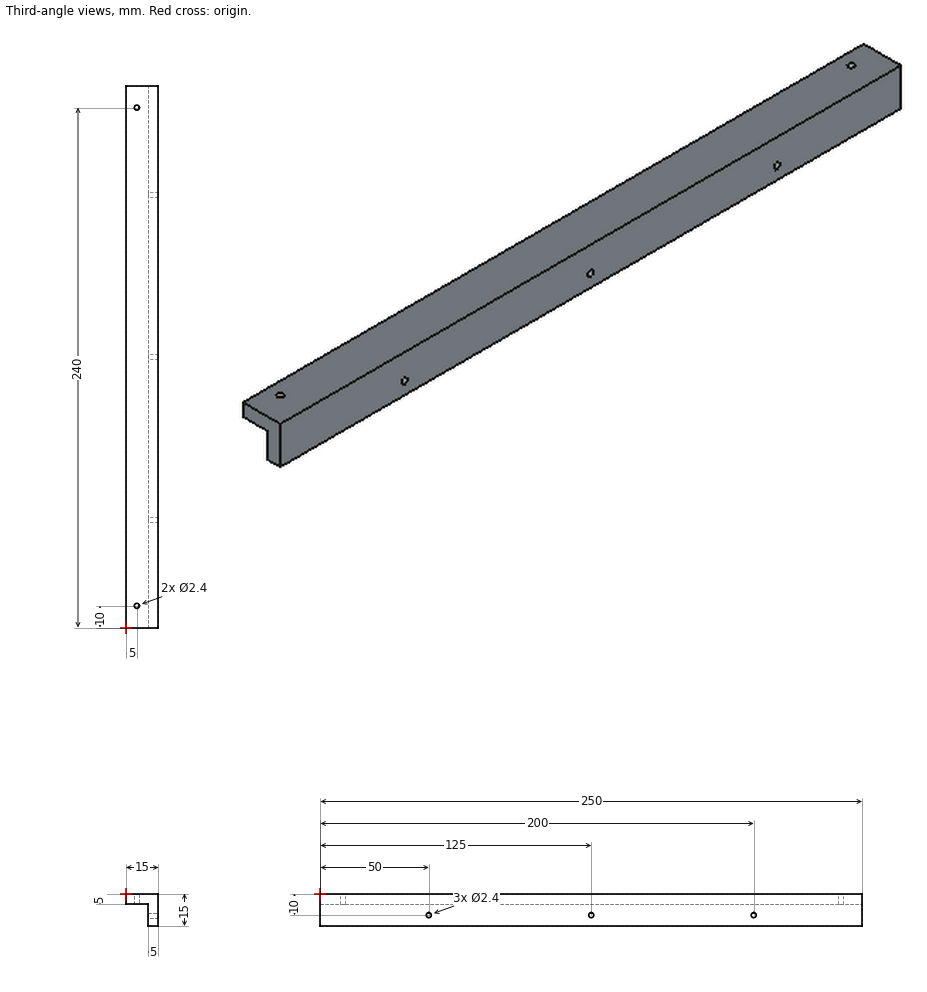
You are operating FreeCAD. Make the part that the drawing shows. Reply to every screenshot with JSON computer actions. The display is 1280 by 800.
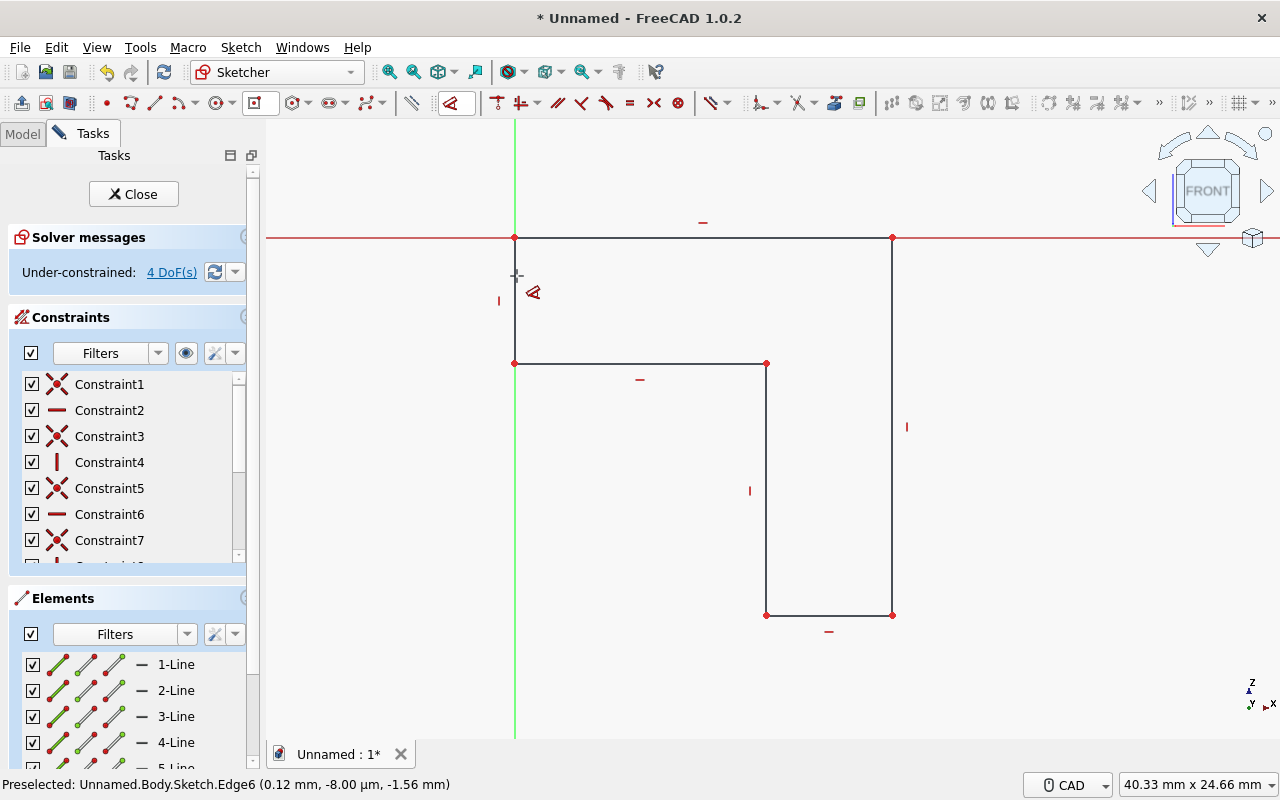
{"action": "left_click", "coordinate": [854, 616]}
{"action": "left_click", "coordinate": [829, 650]}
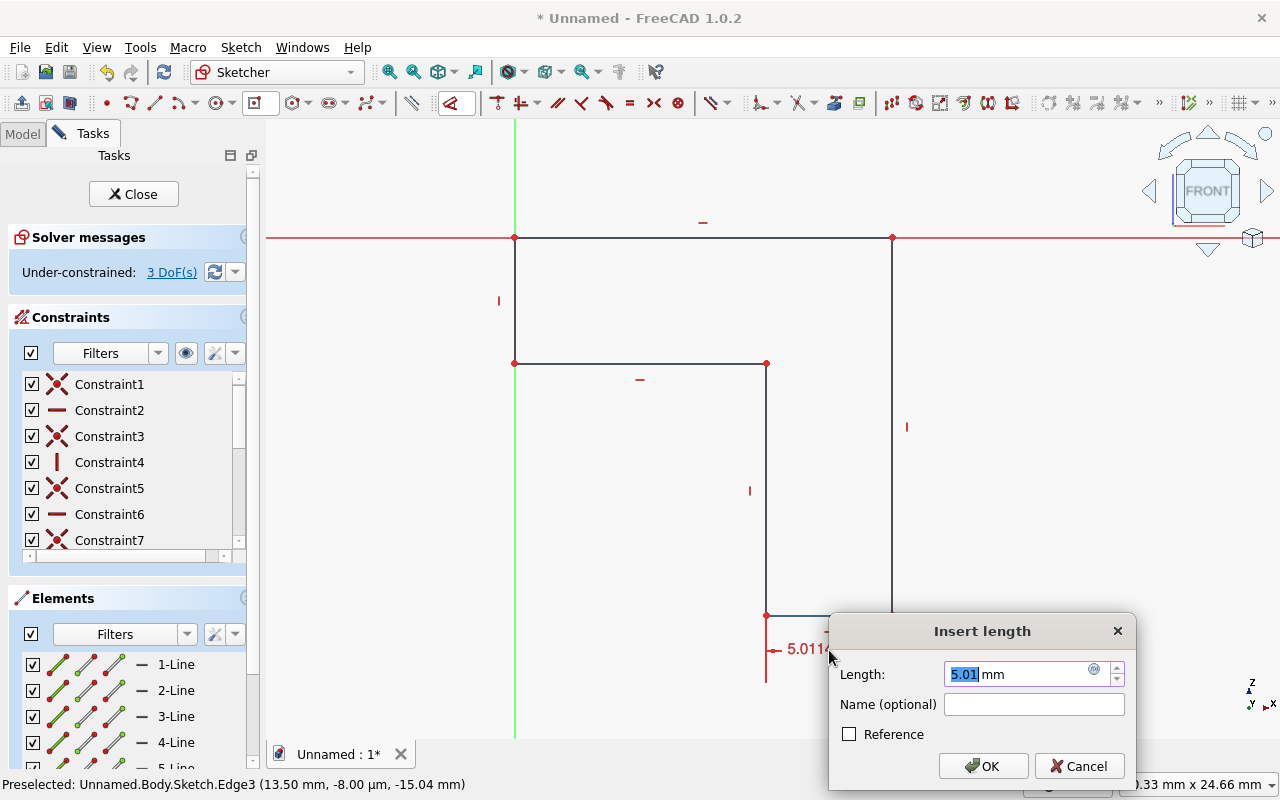
{"action": "type", "text": "5"}
{"action": "key", "text": "Return"}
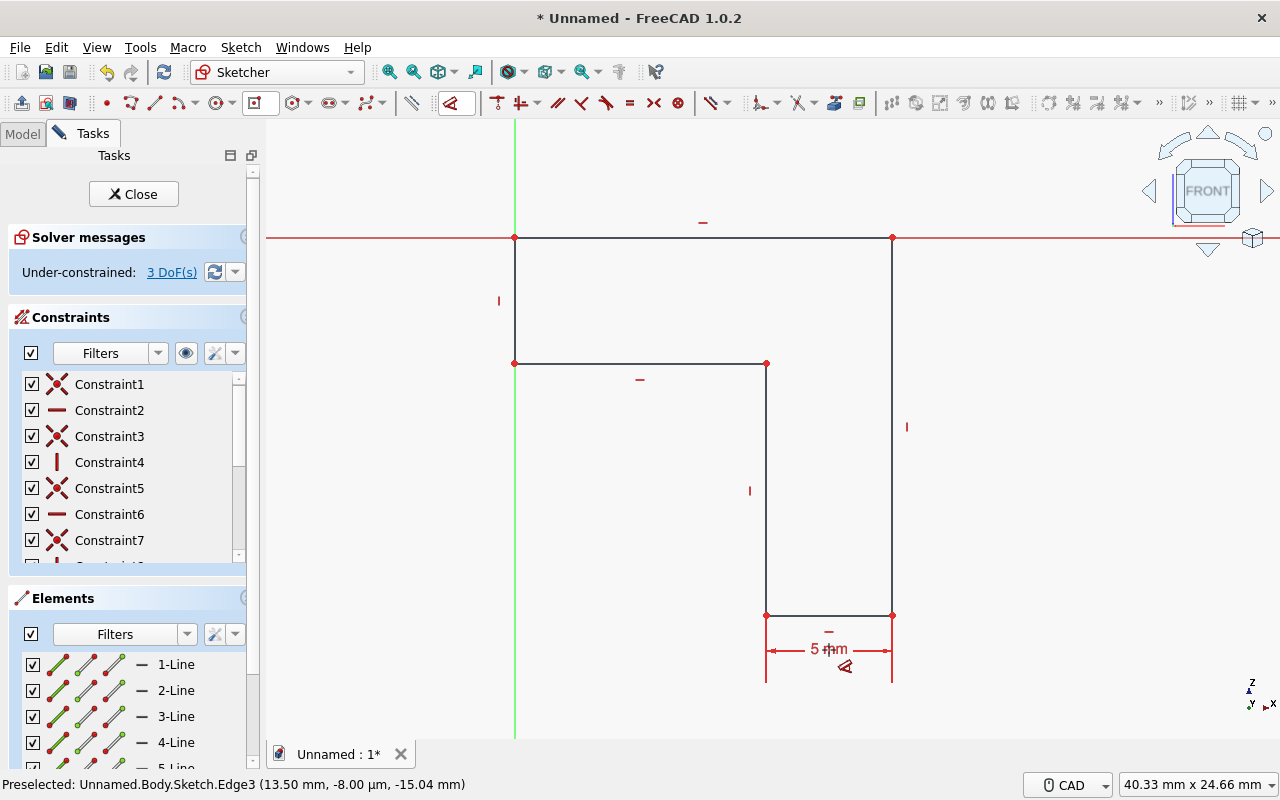
{"action": "left_click", "coordinate": [515, 326]}
{"action": "left_click", "coordinate": [481, 301]}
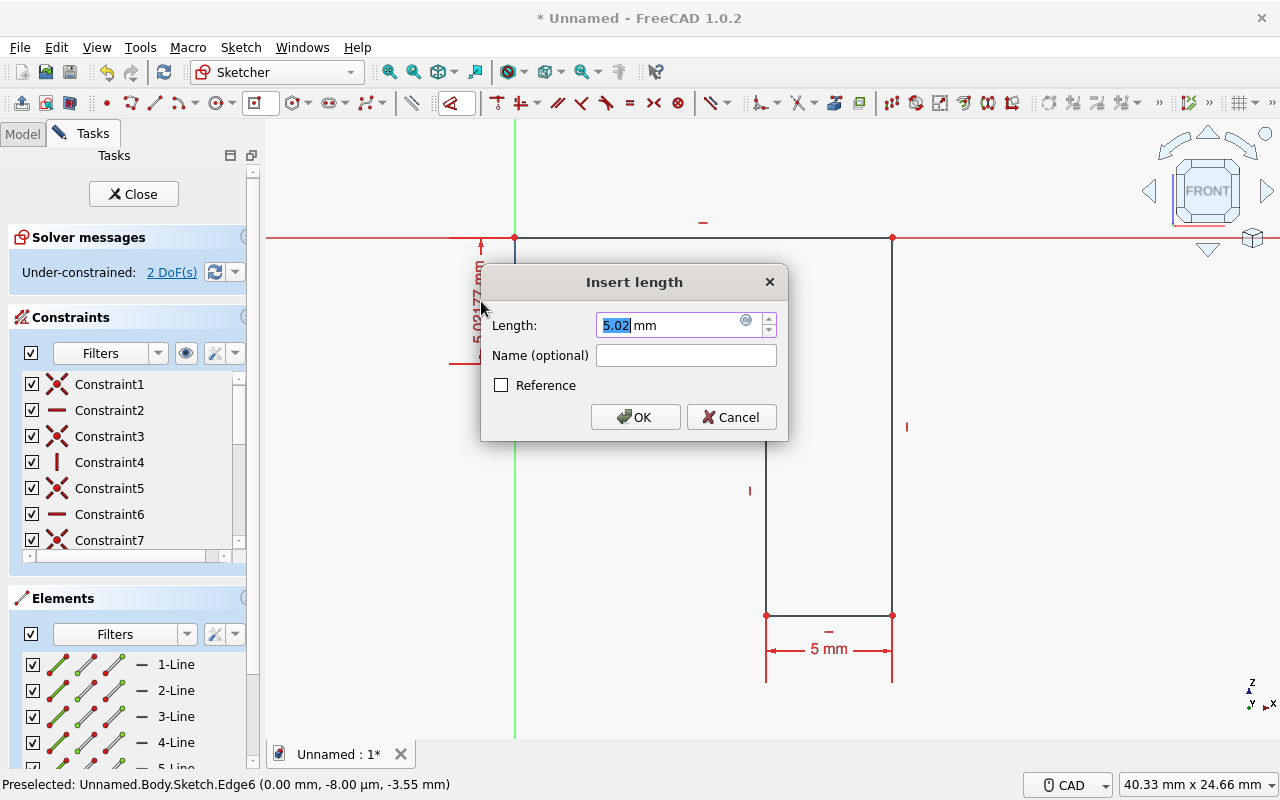
{"action": "type", "text": "5"}
{"action": "key", "text": "Return"}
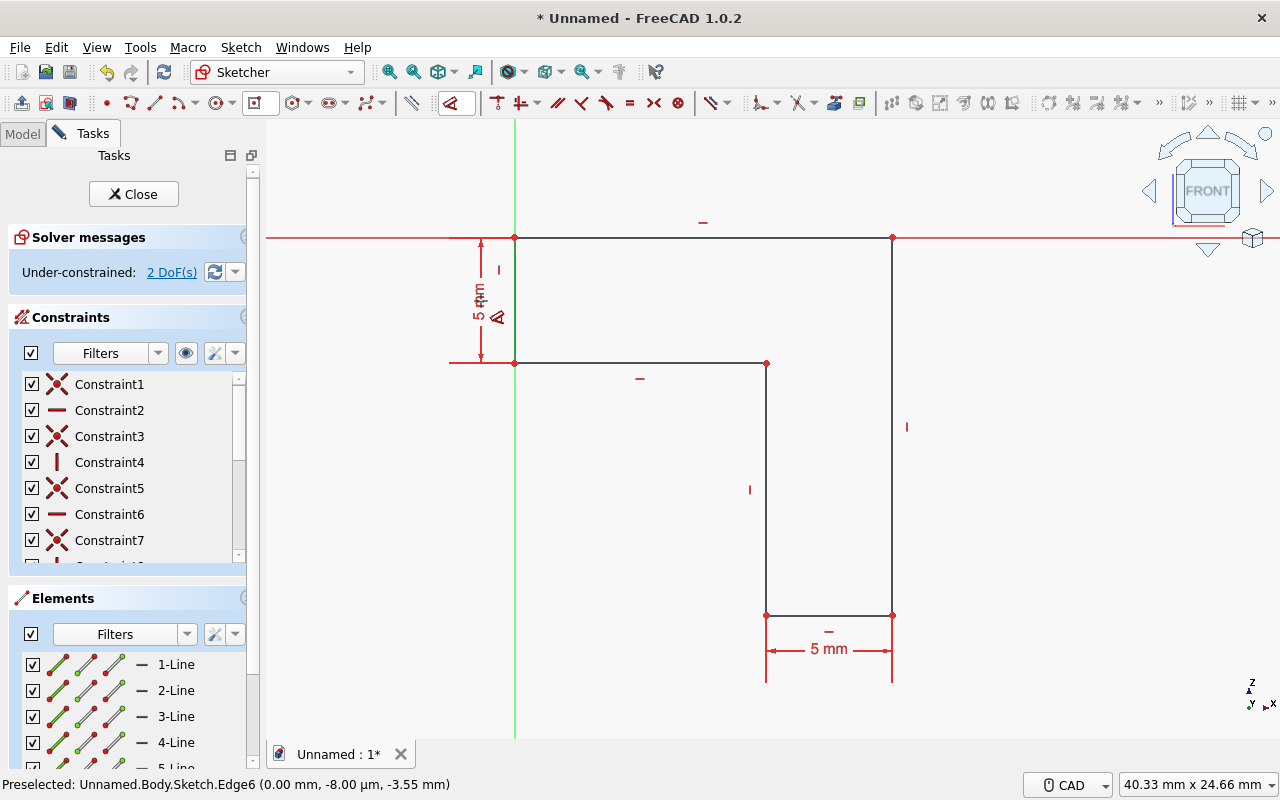
{"action": "left_click", "coordinate": [628, 238]}
{"action": "left_click", "coordinate": [703, 204]}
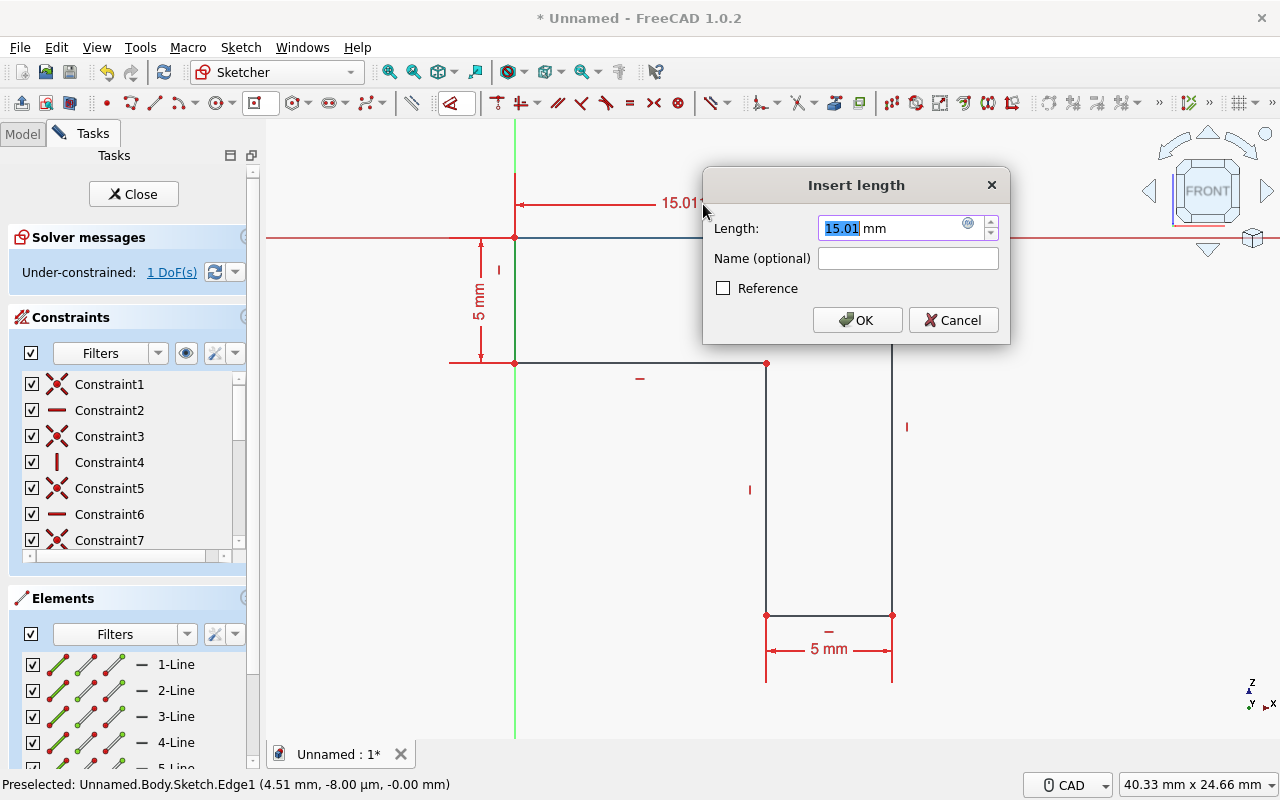
{"action": "type", "text": "15"}
{"action": "key", "text": "Return"}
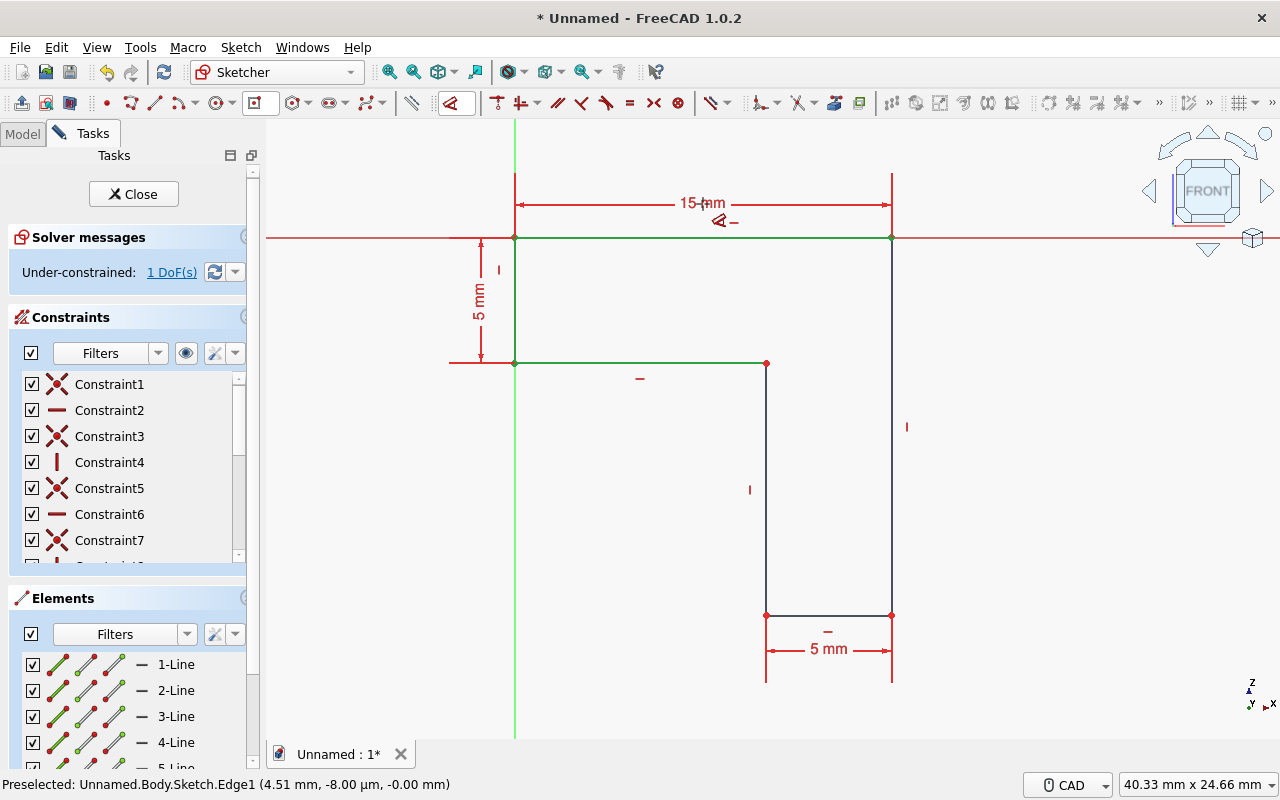
{"action": "left_click", "coordinate": [892, 351]}
{"action": "left_click", "coordinate": [926, 427]}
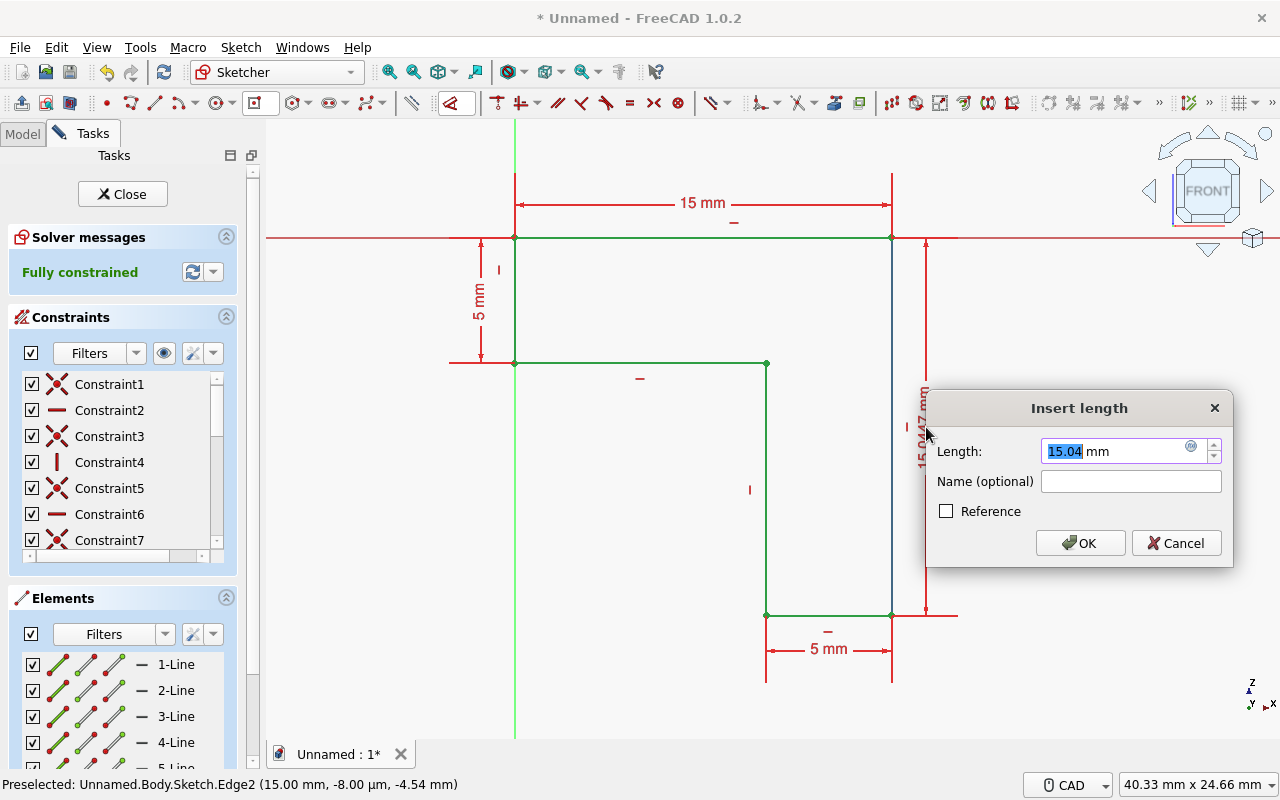
{"action": "type", "text": "15"}
{"action": "key", "text": "Return"}
{"action": "key", "text": "Escape"}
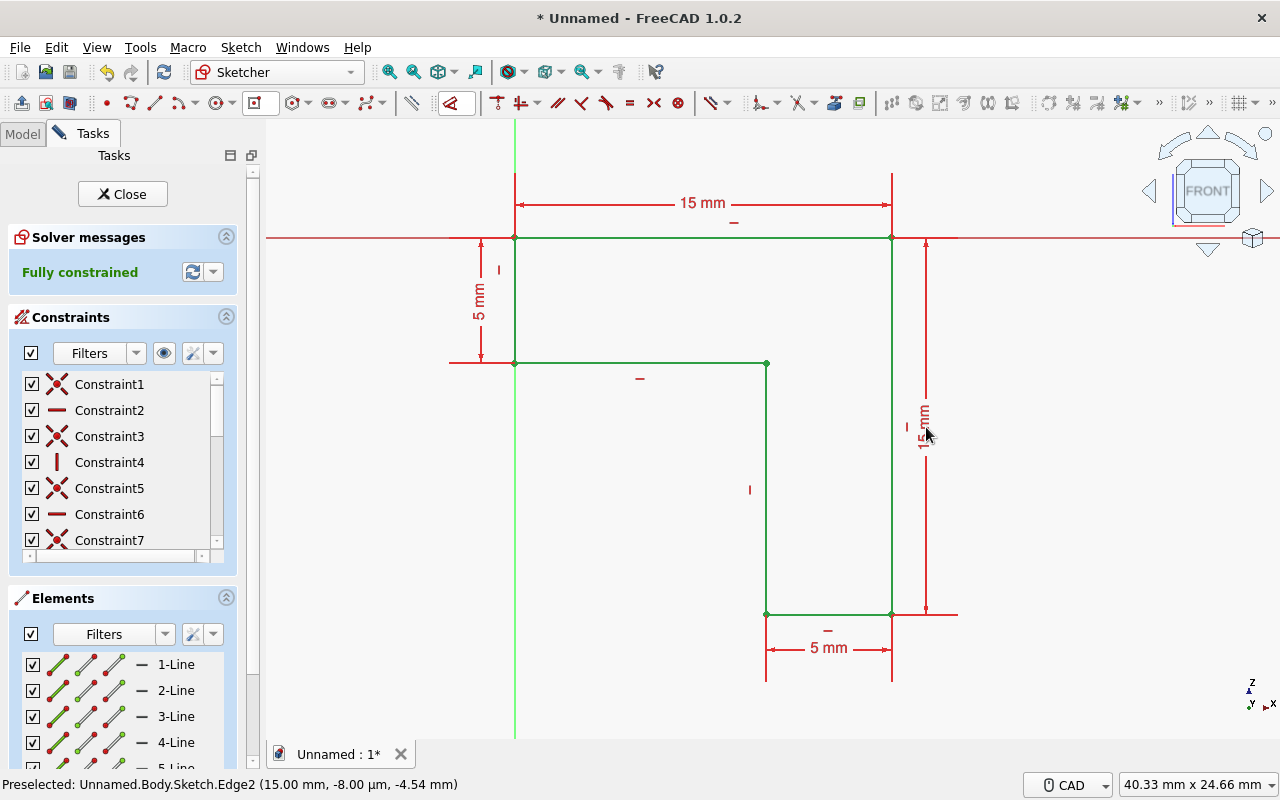
{"action": "left_click", "coordinate": [123, 194]}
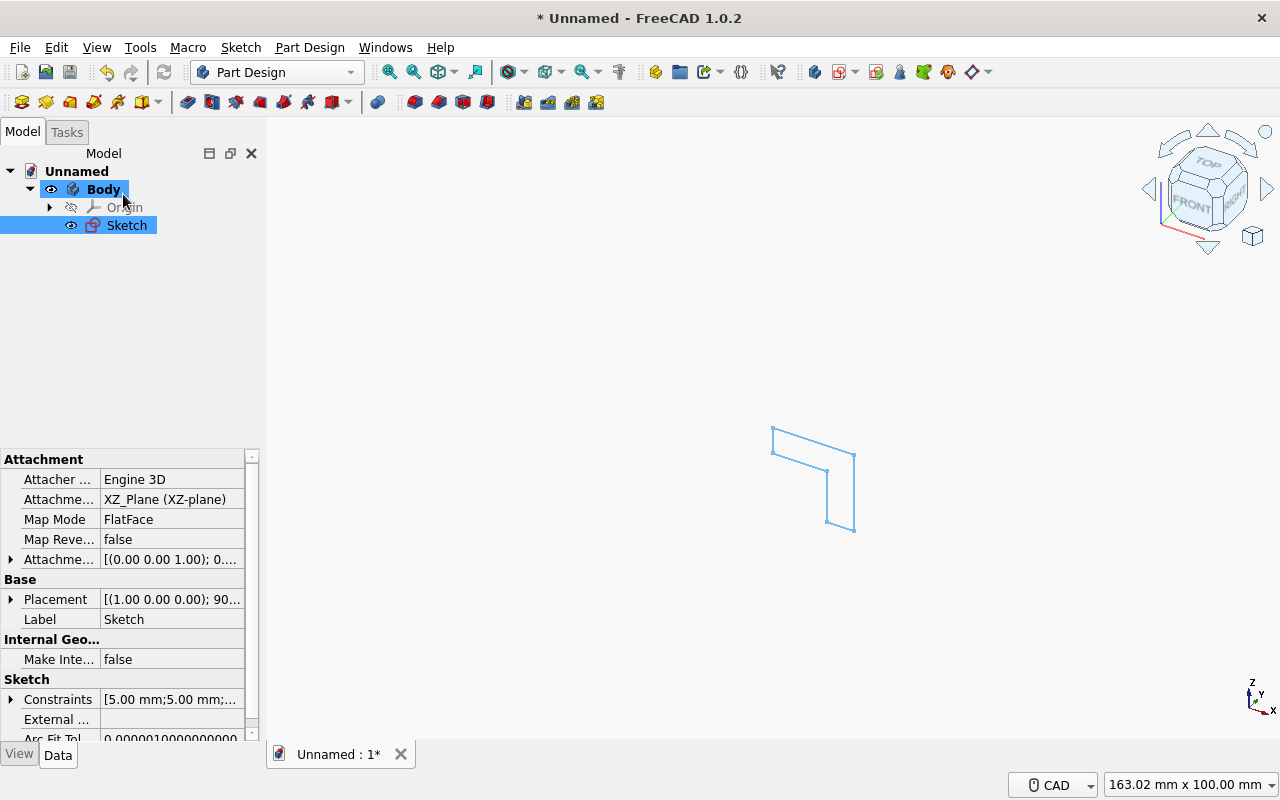
{"action": "left_click", "coordinate": [22, 102]}